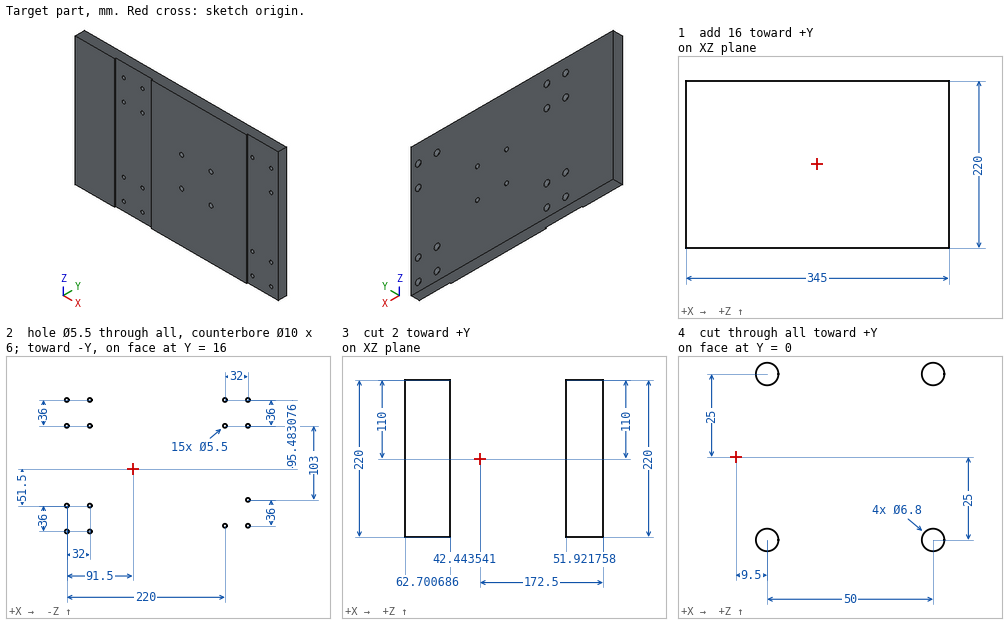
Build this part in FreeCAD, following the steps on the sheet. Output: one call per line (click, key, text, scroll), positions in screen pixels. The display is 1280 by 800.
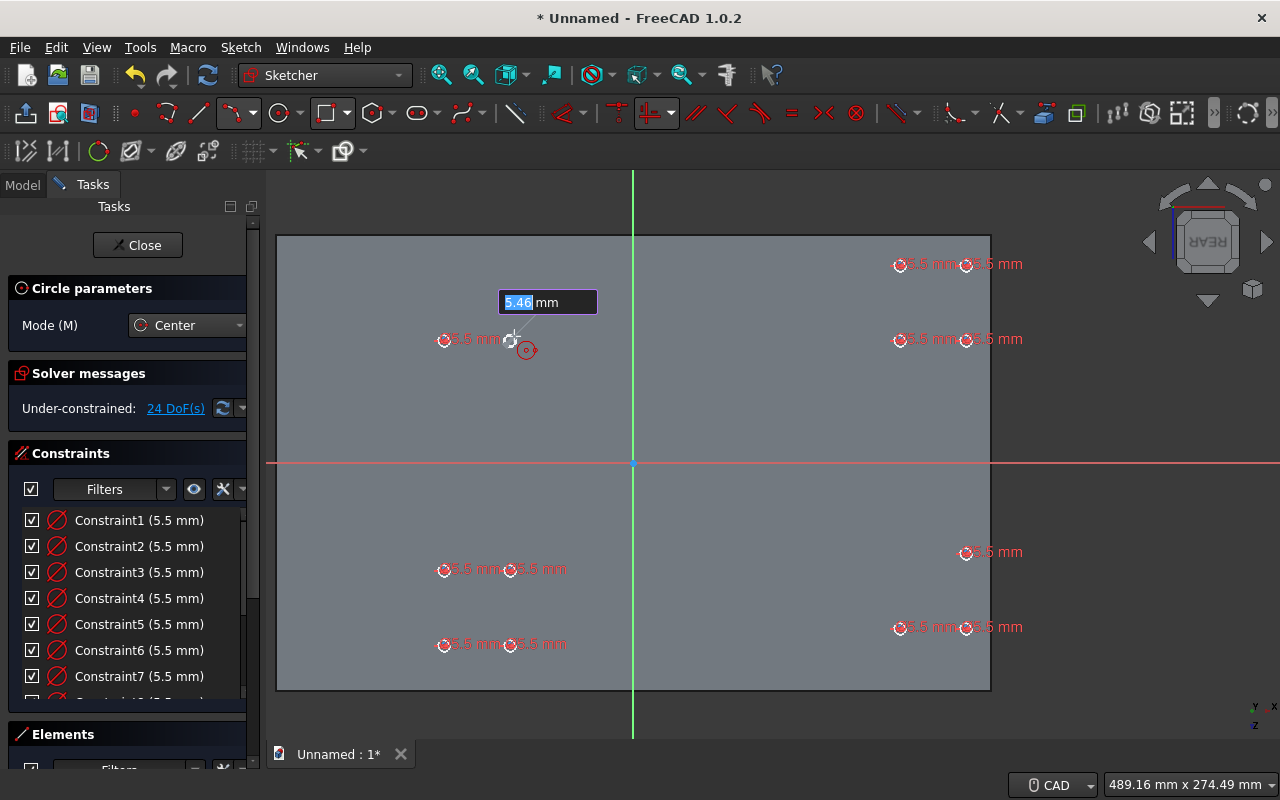
text(5.5)
key(Return)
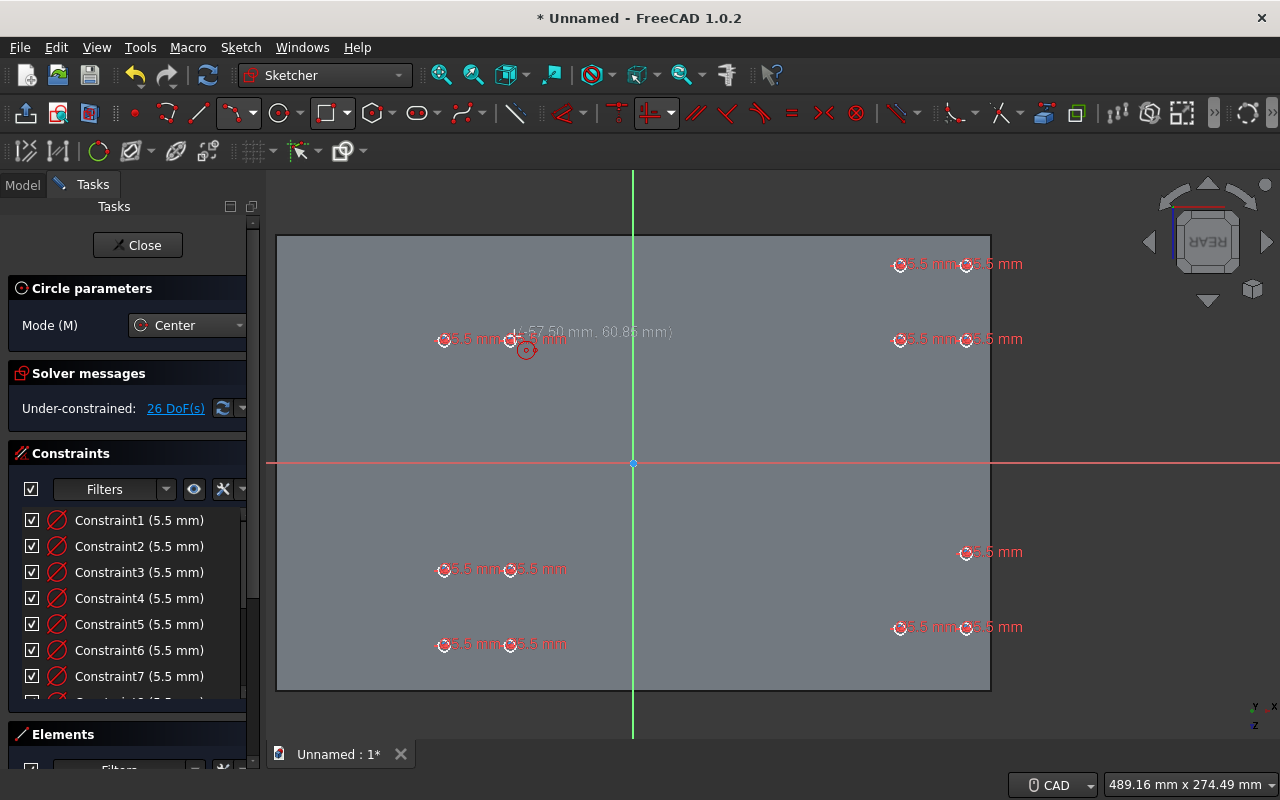
scroll(510, 265, up, 7)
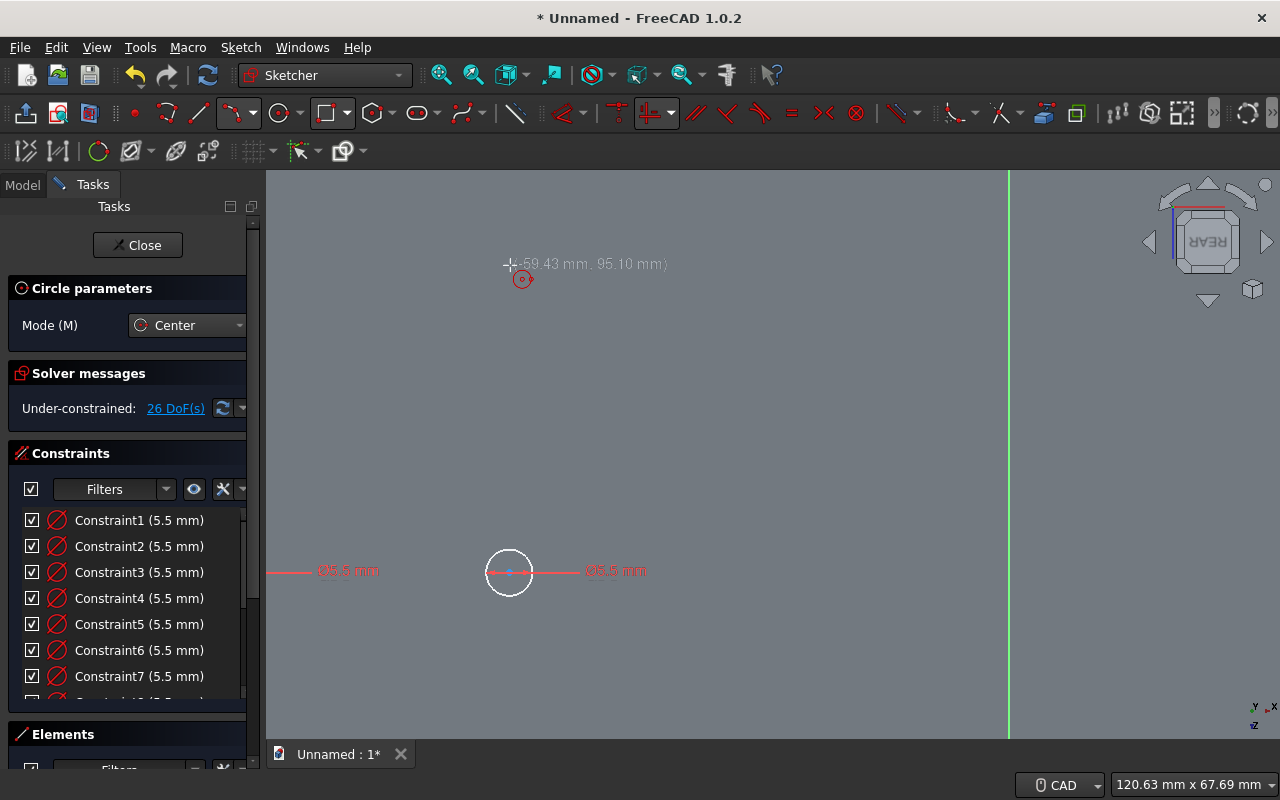
scroll(510, 265, down, 7)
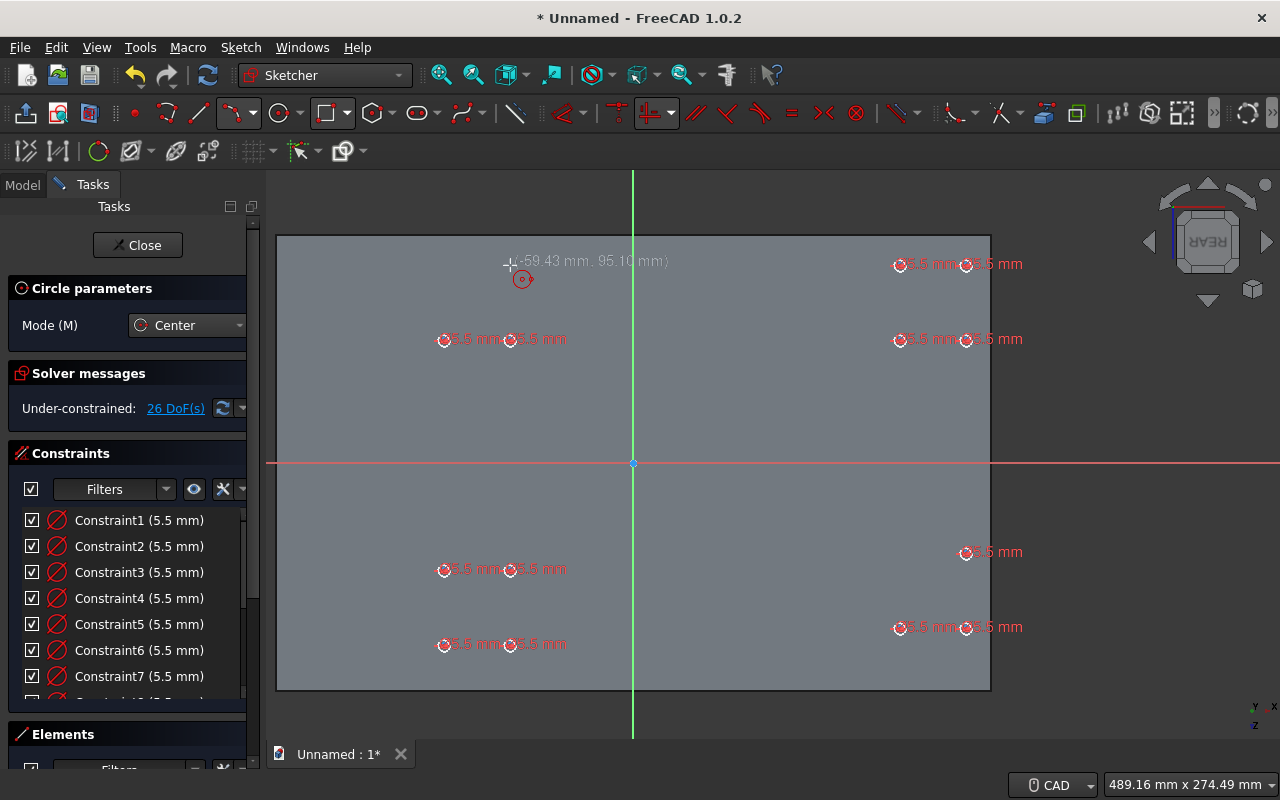
click(510, 265)
move(514, 261)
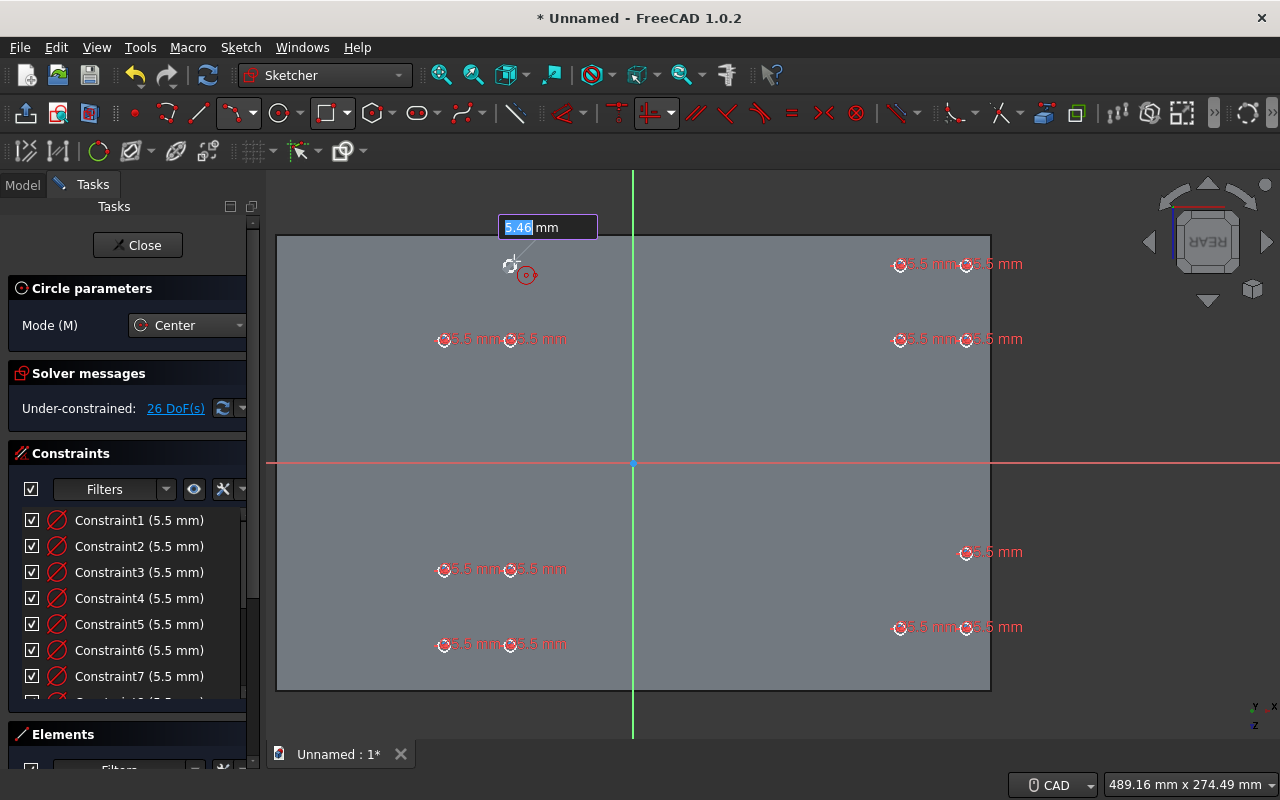
text(5.5)
key(Return)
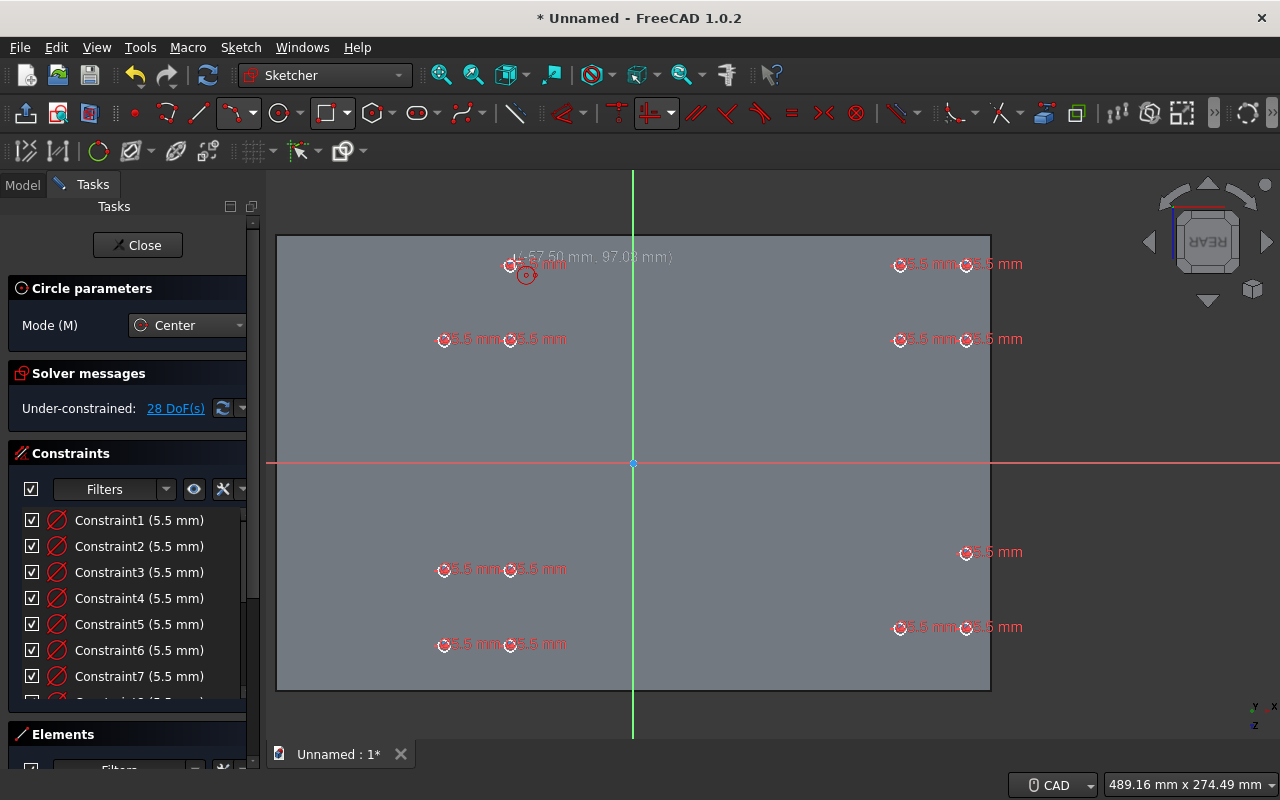
scroll(444, 265, up, 7)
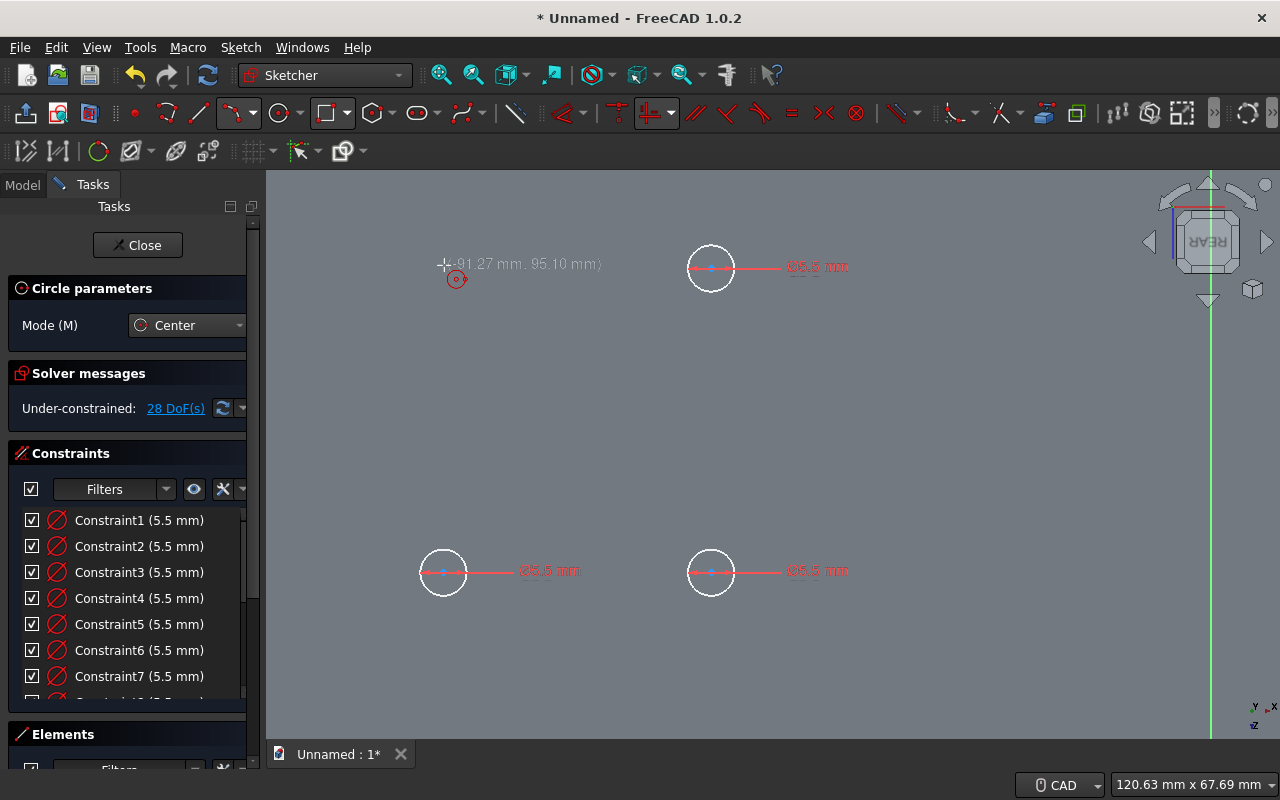
scroll(444, 265, down, 7)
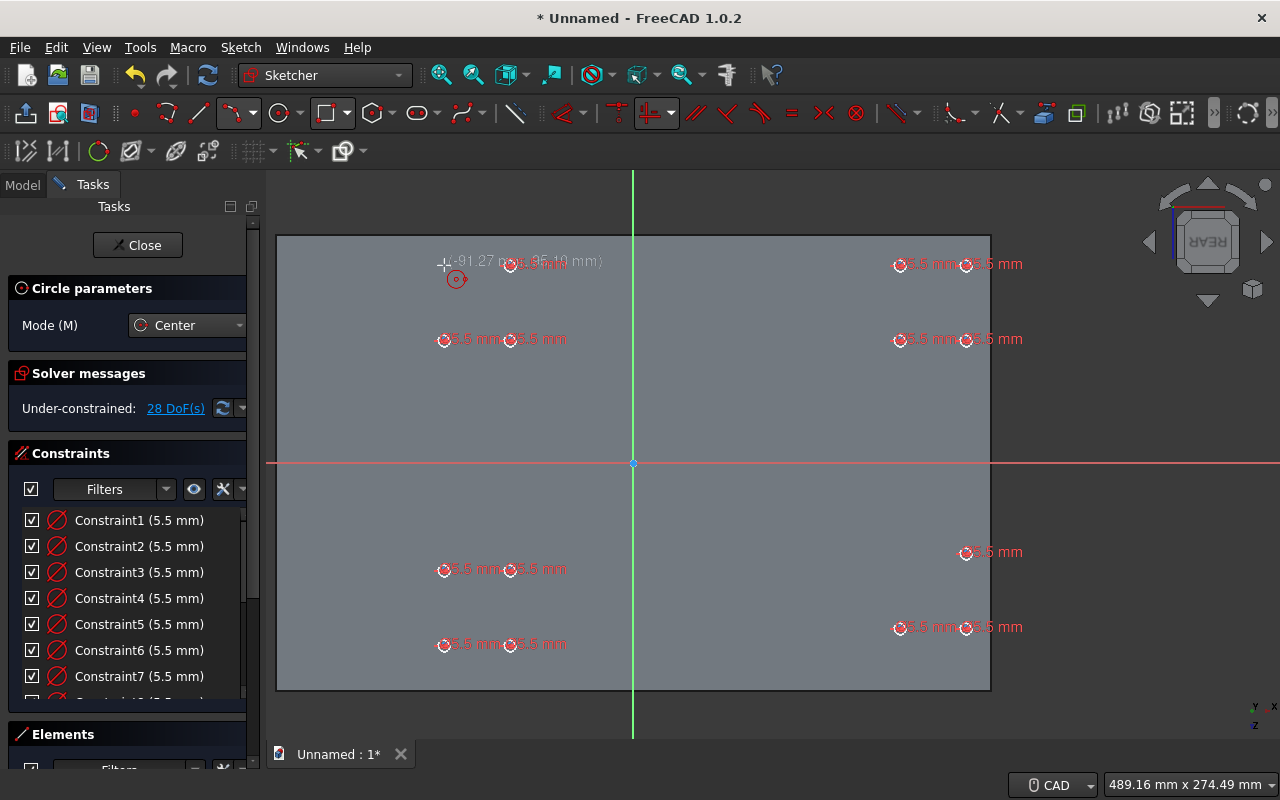
click(444, 265)
move(448, 261)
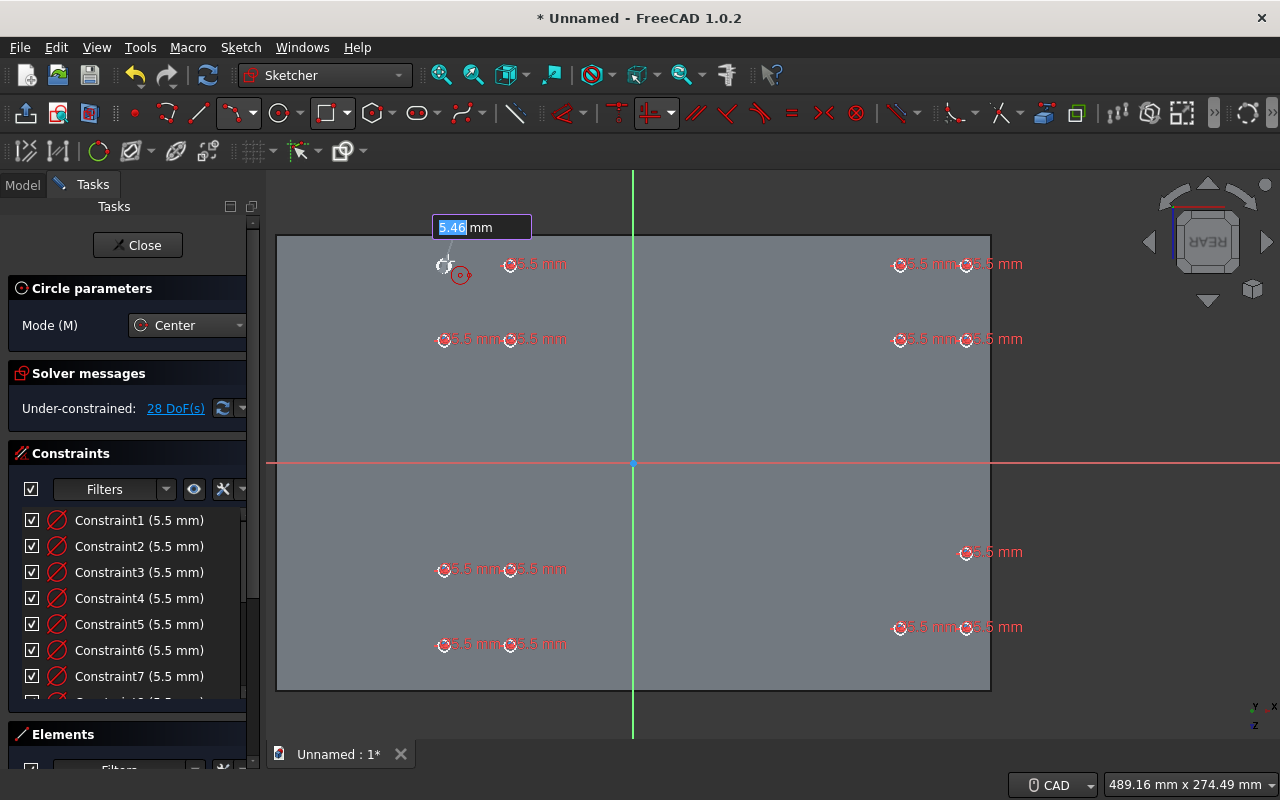
text(5.5)
key(Return)
key(Escape)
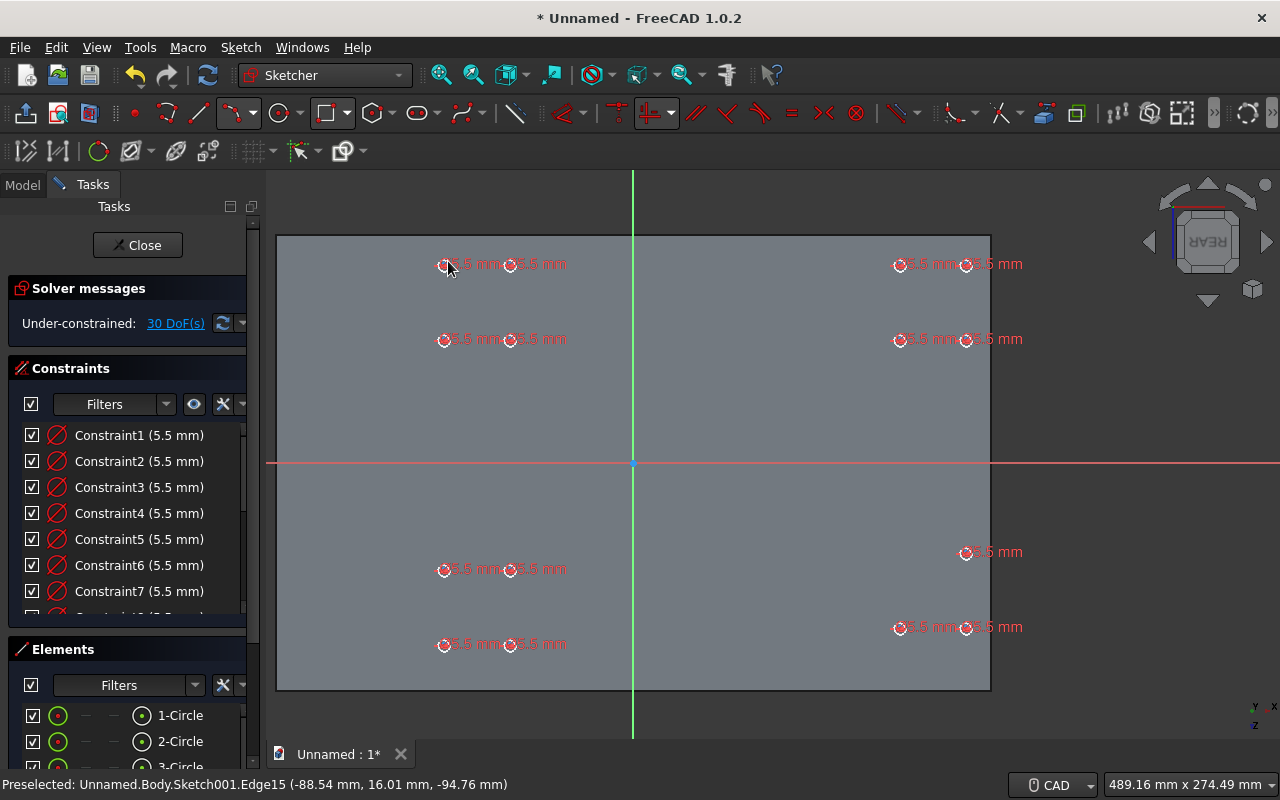
click(966, 266)